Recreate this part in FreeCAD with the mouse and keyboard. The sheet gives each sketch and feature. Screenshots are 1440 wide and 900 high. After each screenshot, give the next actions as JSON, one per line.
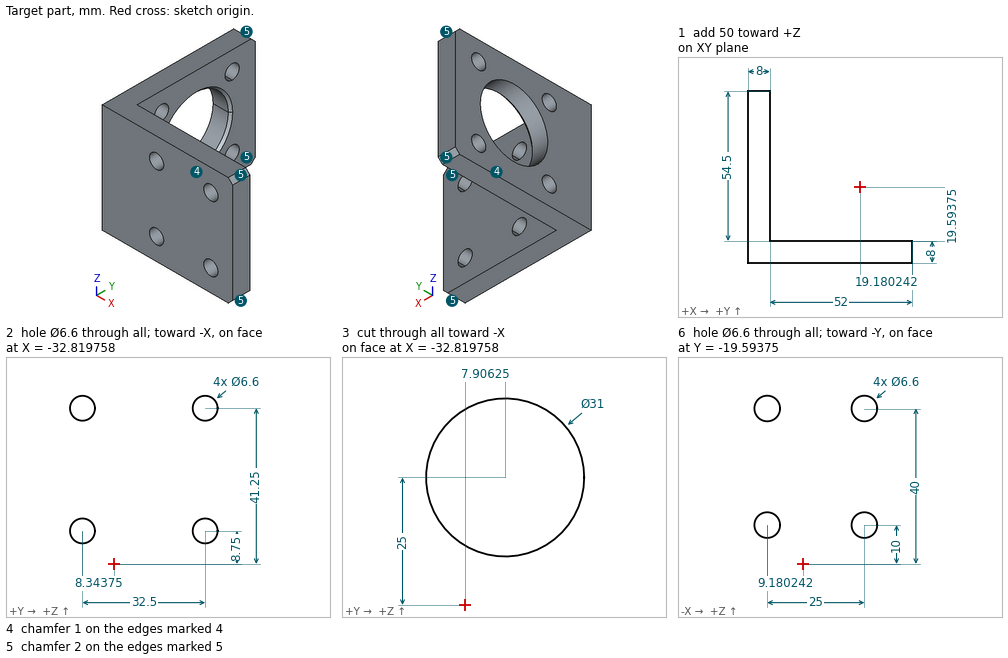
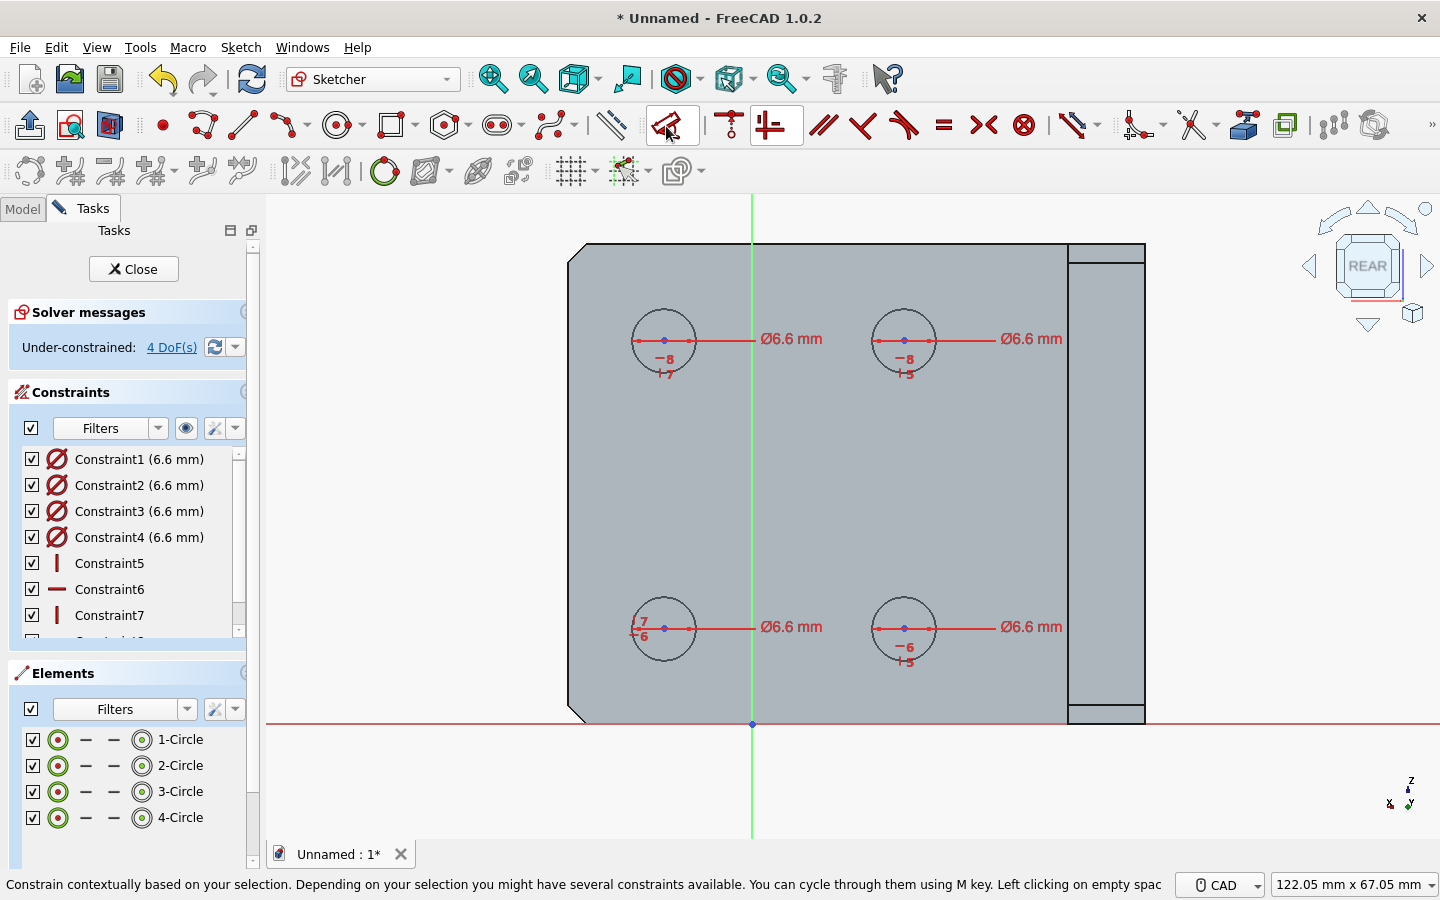
{"action": "left_click", "coordinate": [904, 341]}
{"action": "left_click", "coordinate": [938, 533]}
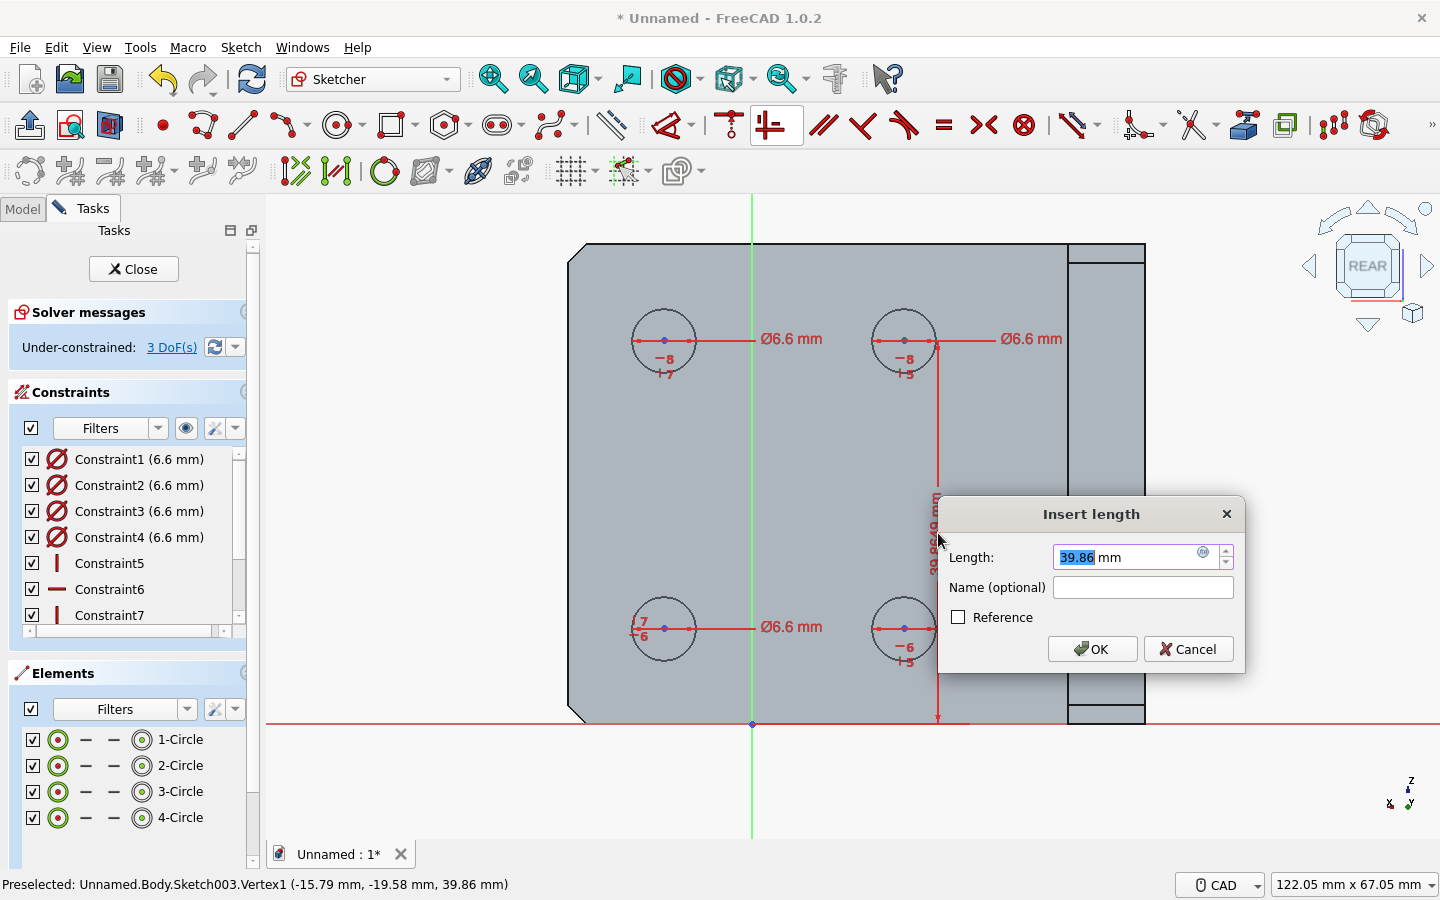
{"action": "type", "text": "40"}
{"action": "key", "text": "Return"}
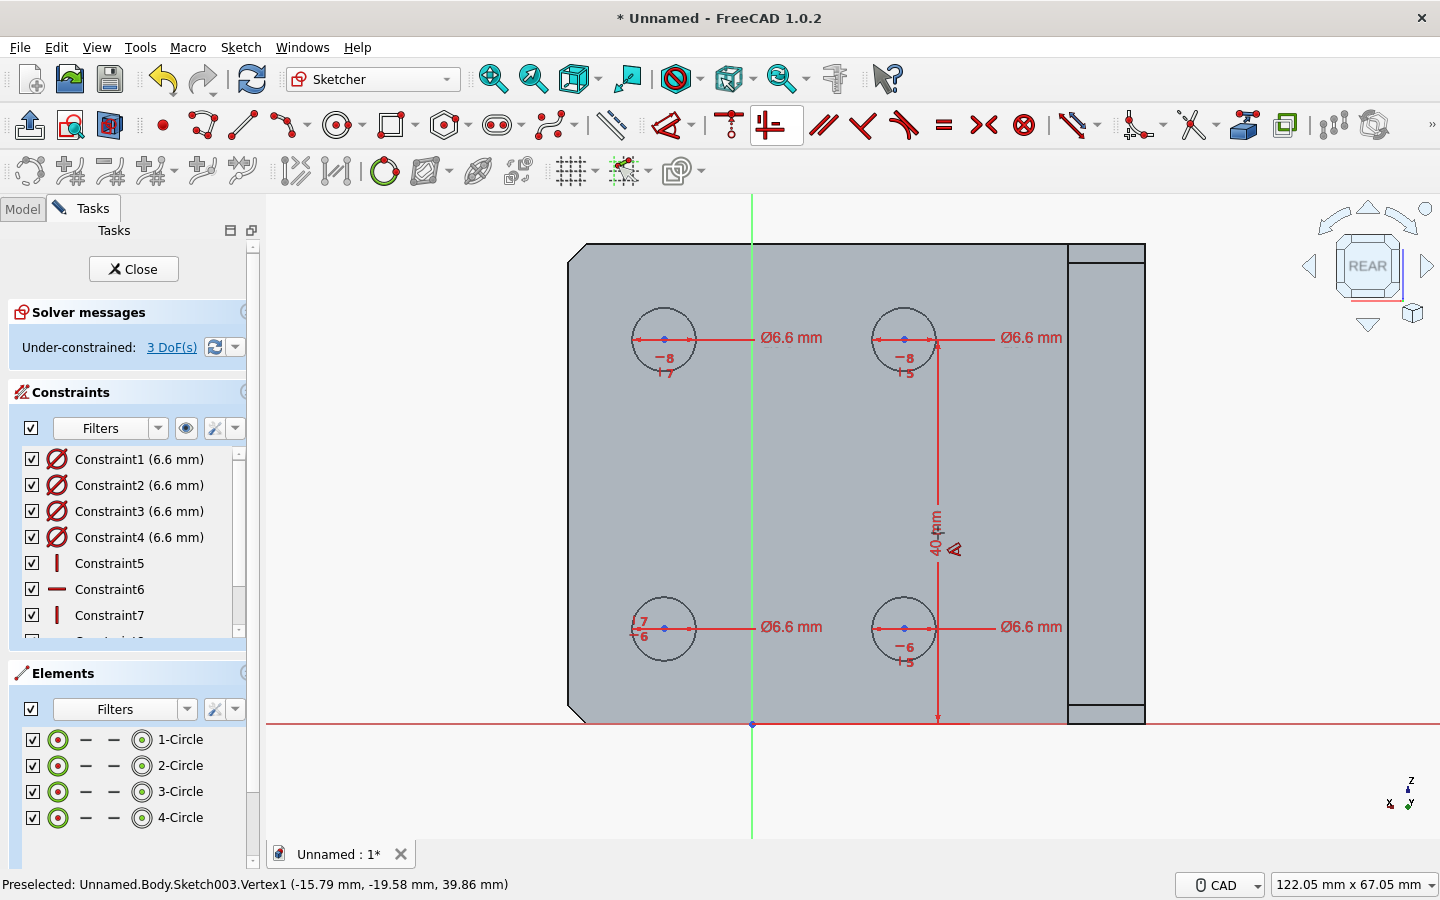
{"action": "left_click", "coordinate": [904, 629]}
{"action": "left_click", "coordinate": [938, 677]}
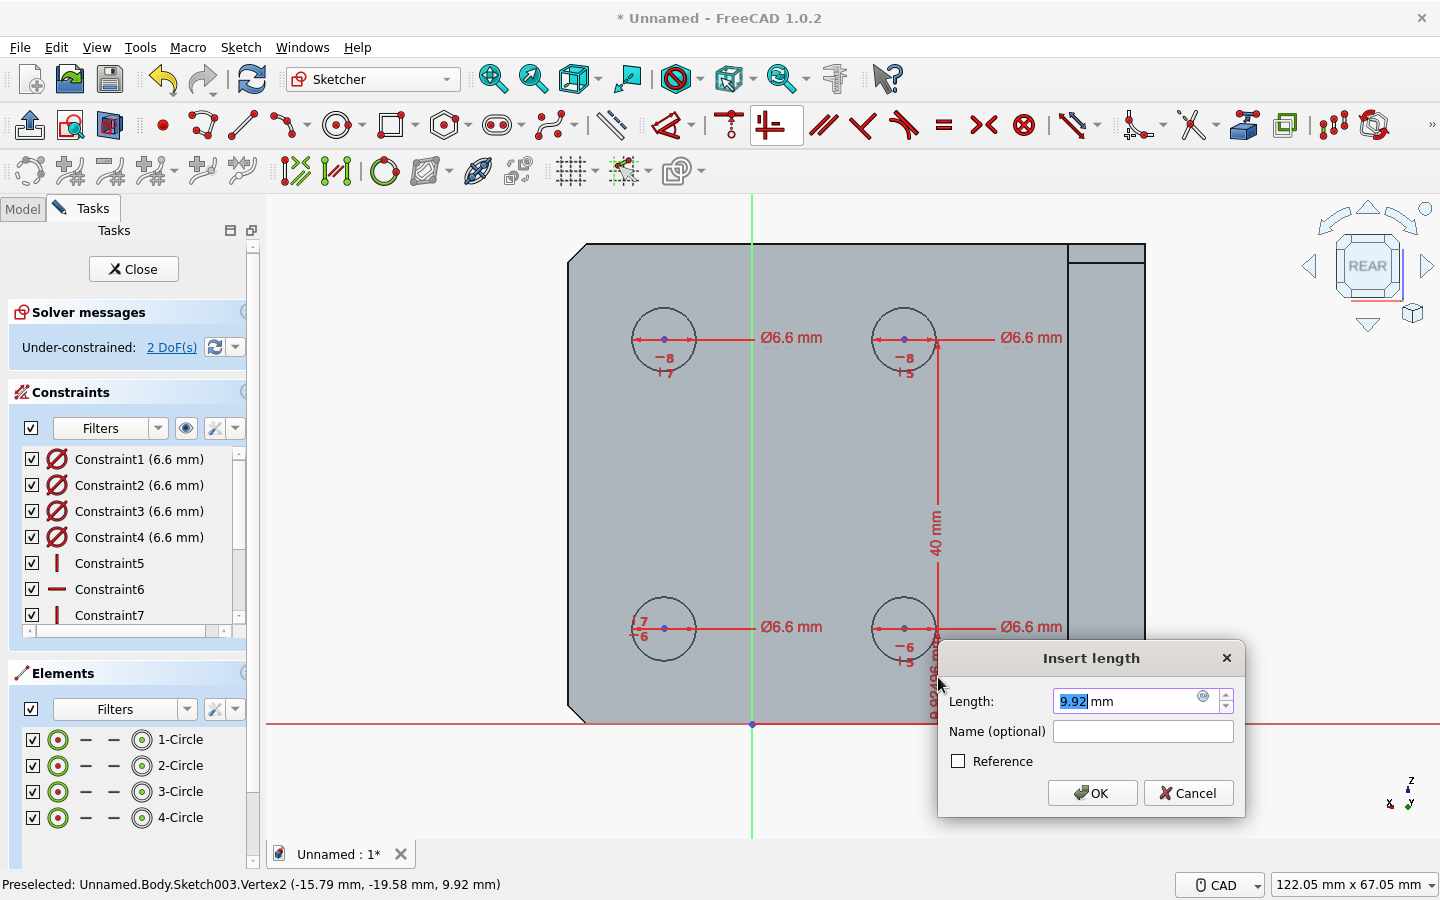
{"action": "type", "text": "10"}
{"action": "key", "text": "Return"}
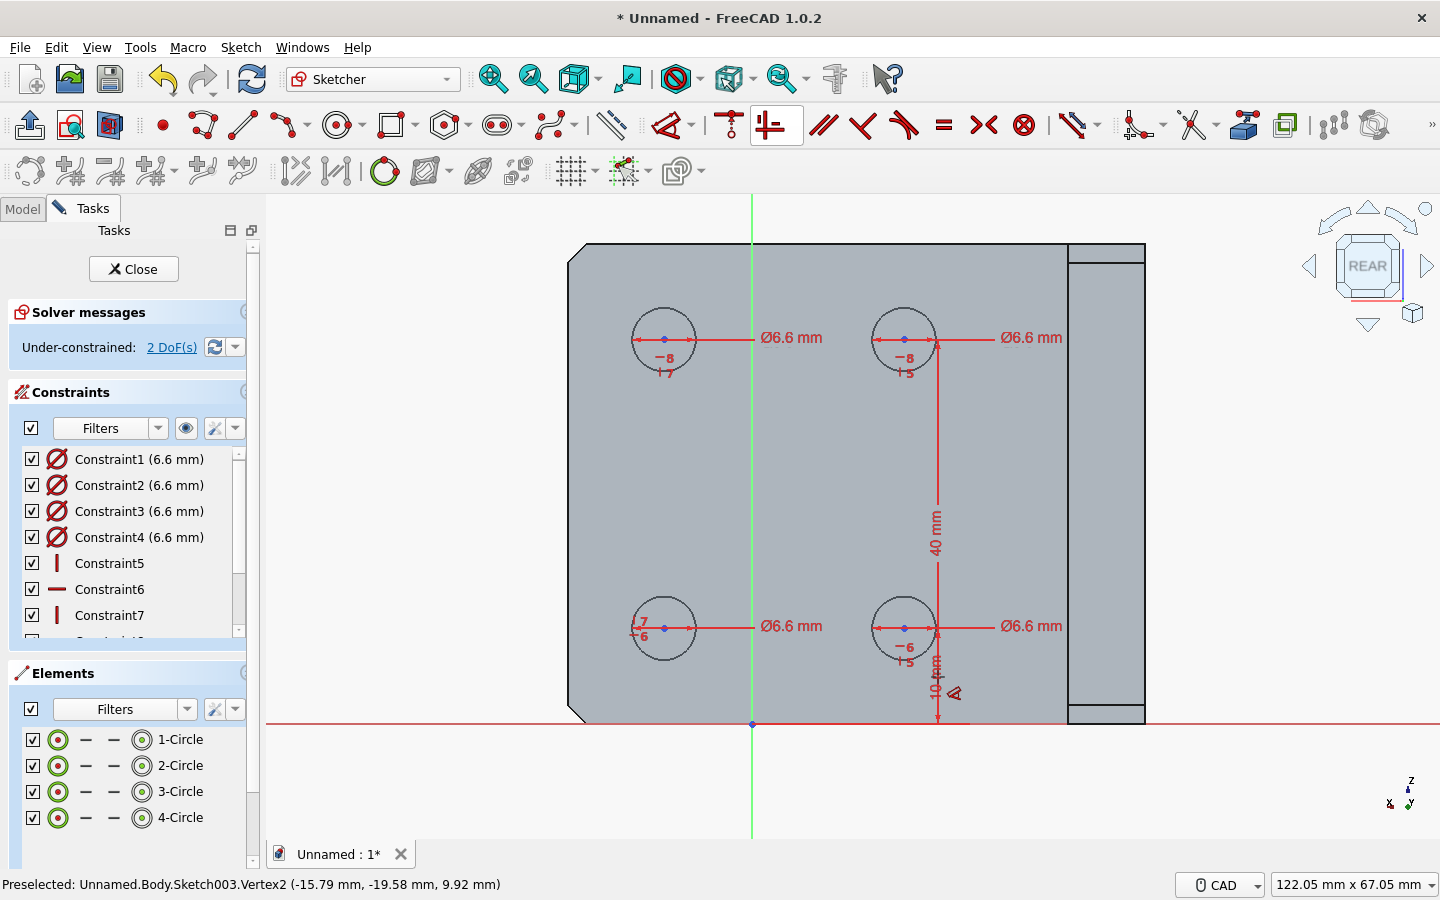
{"action": "left_click", "coordinate": [904, 628]}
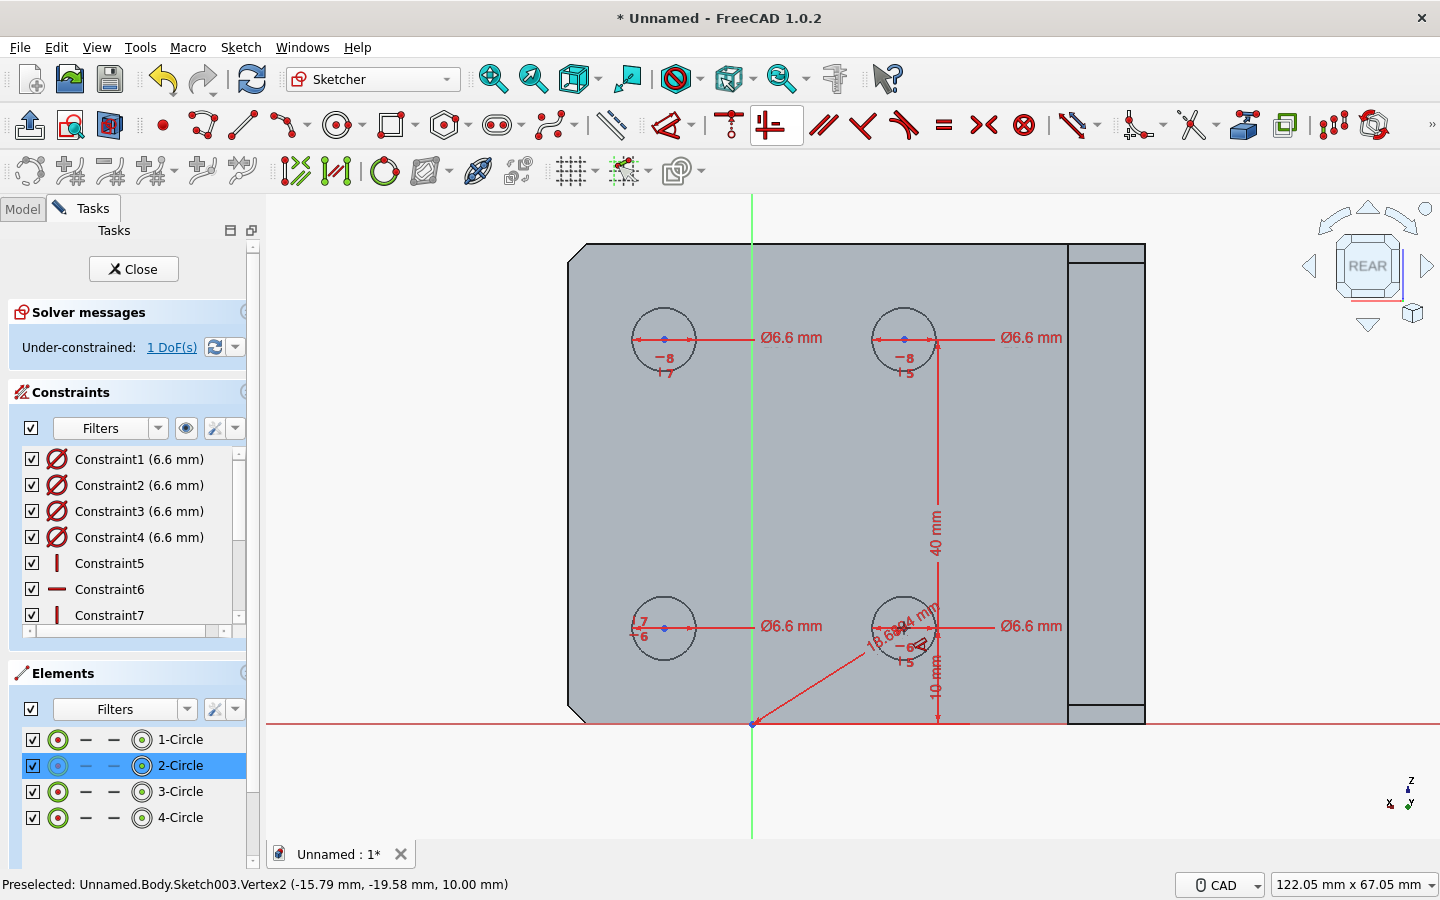
{"action": "left_click", "coordinate": [664, 628]}
{"action": "left_click", "coordinate": [784, 662]}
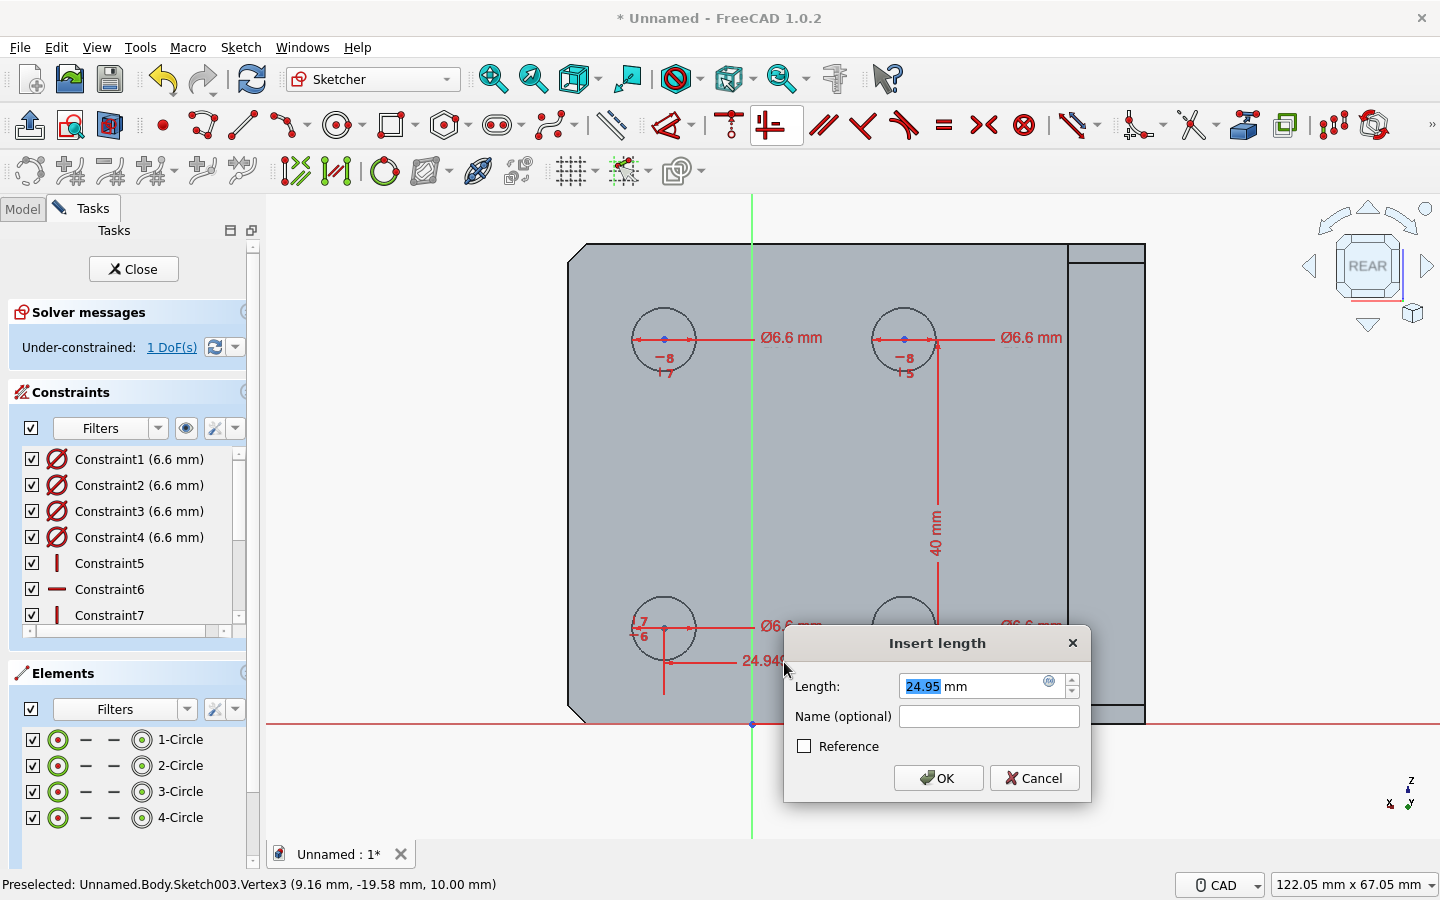
{"action": "type", "text": "25"}
{"action": "key", "text": "Return"}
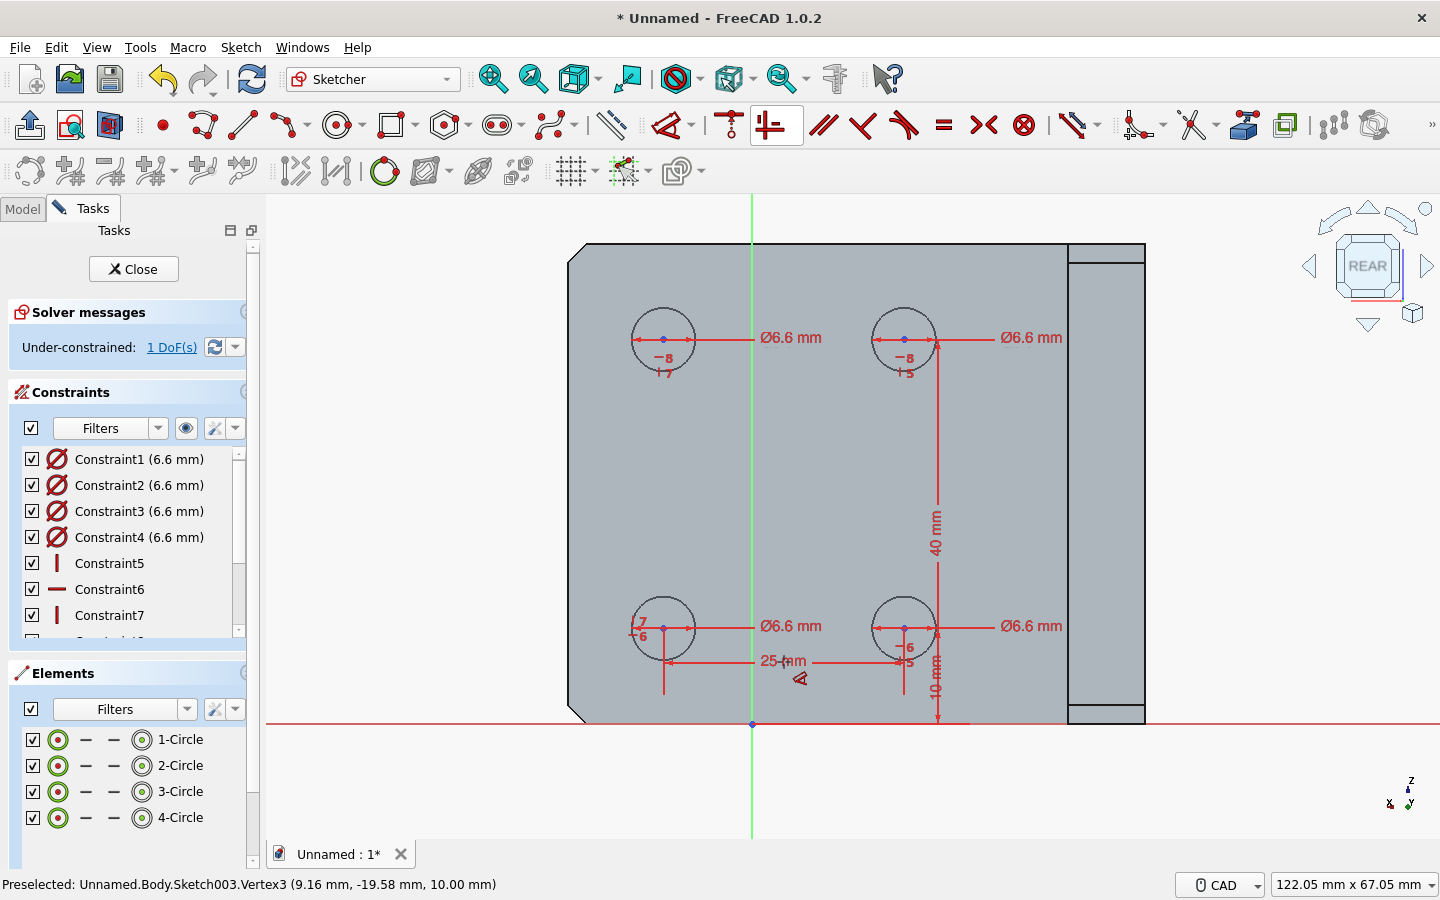
{"action": "left_click", "coordinate": [664, 628]}
{"action": "left_click", "coordinate": [708, 758]}